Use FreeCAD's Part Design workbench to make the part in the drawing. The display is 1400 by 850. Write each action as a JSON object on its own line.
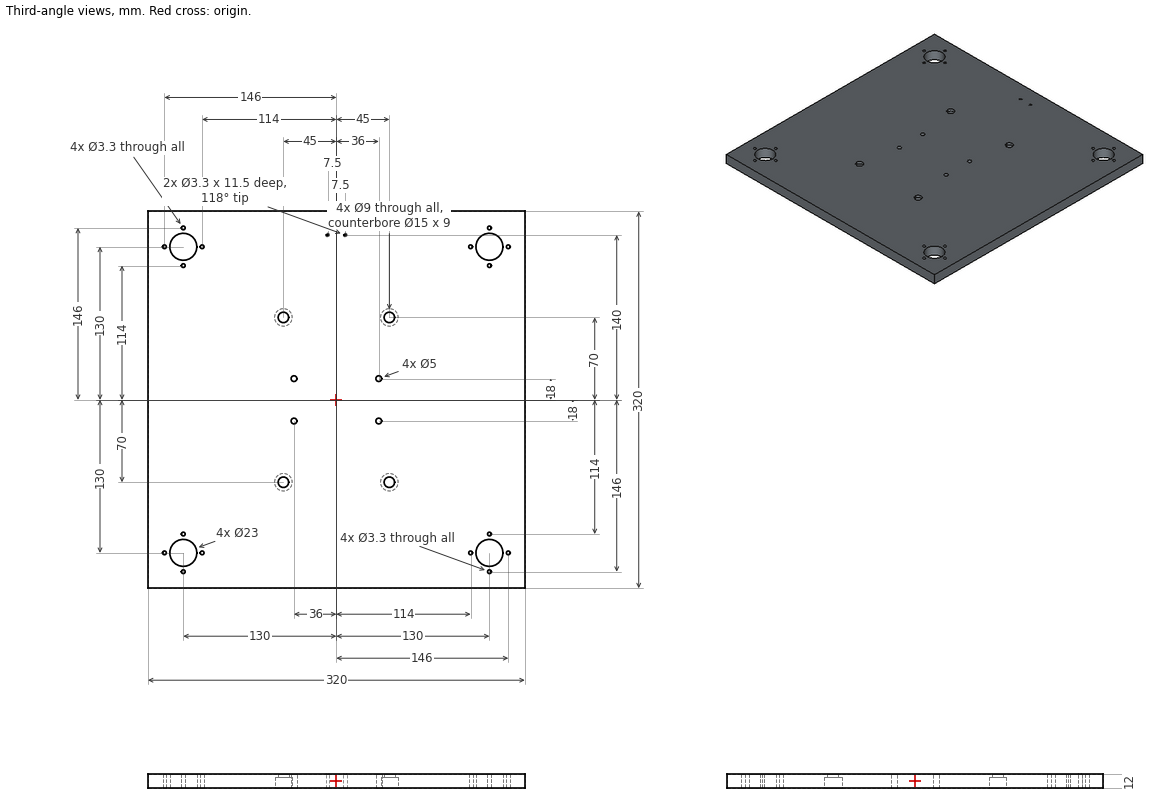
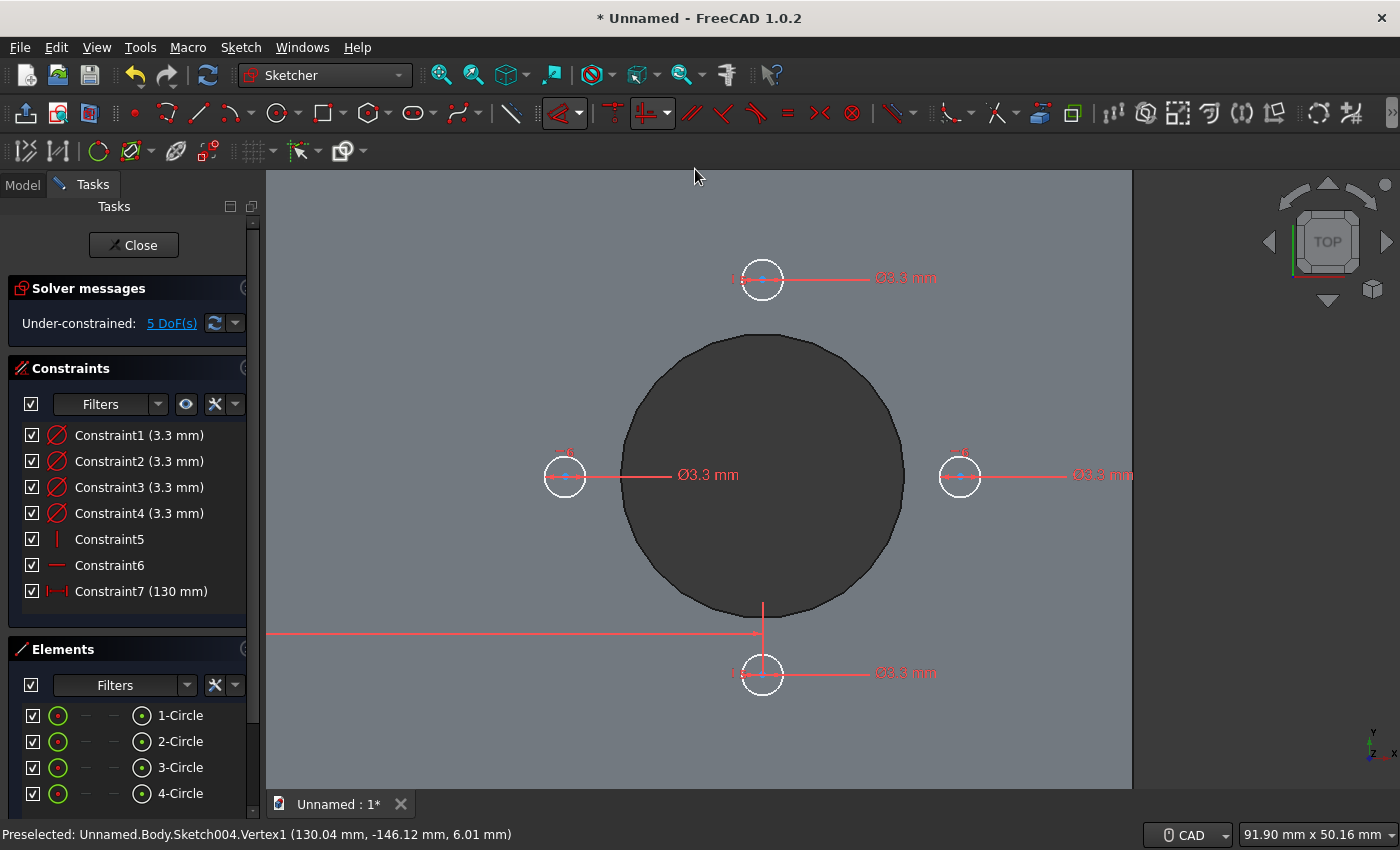
{"action": "left_click", "coordinate": [763, 675]}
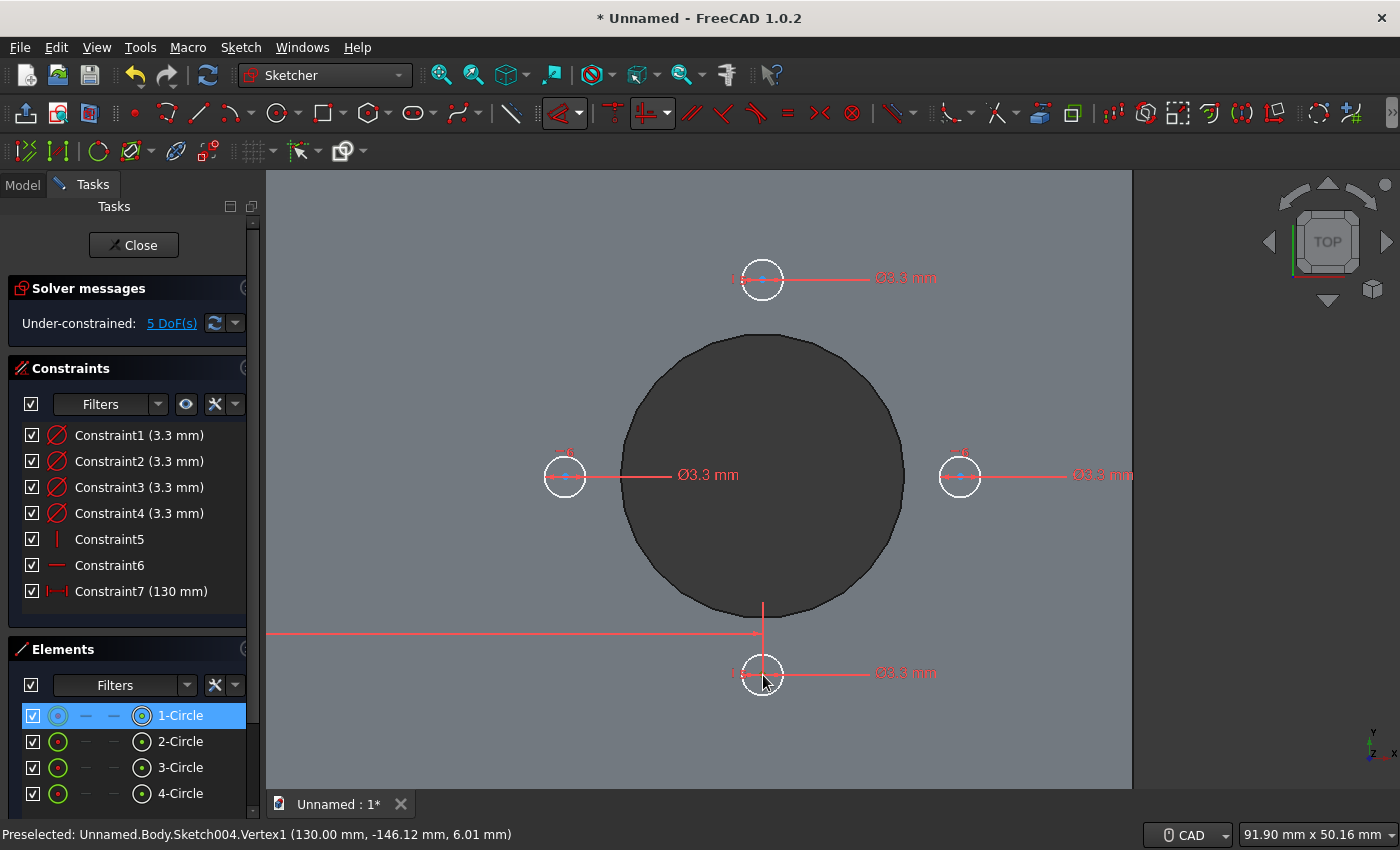
{"action": "left_click", "coordinate": [582, 114]}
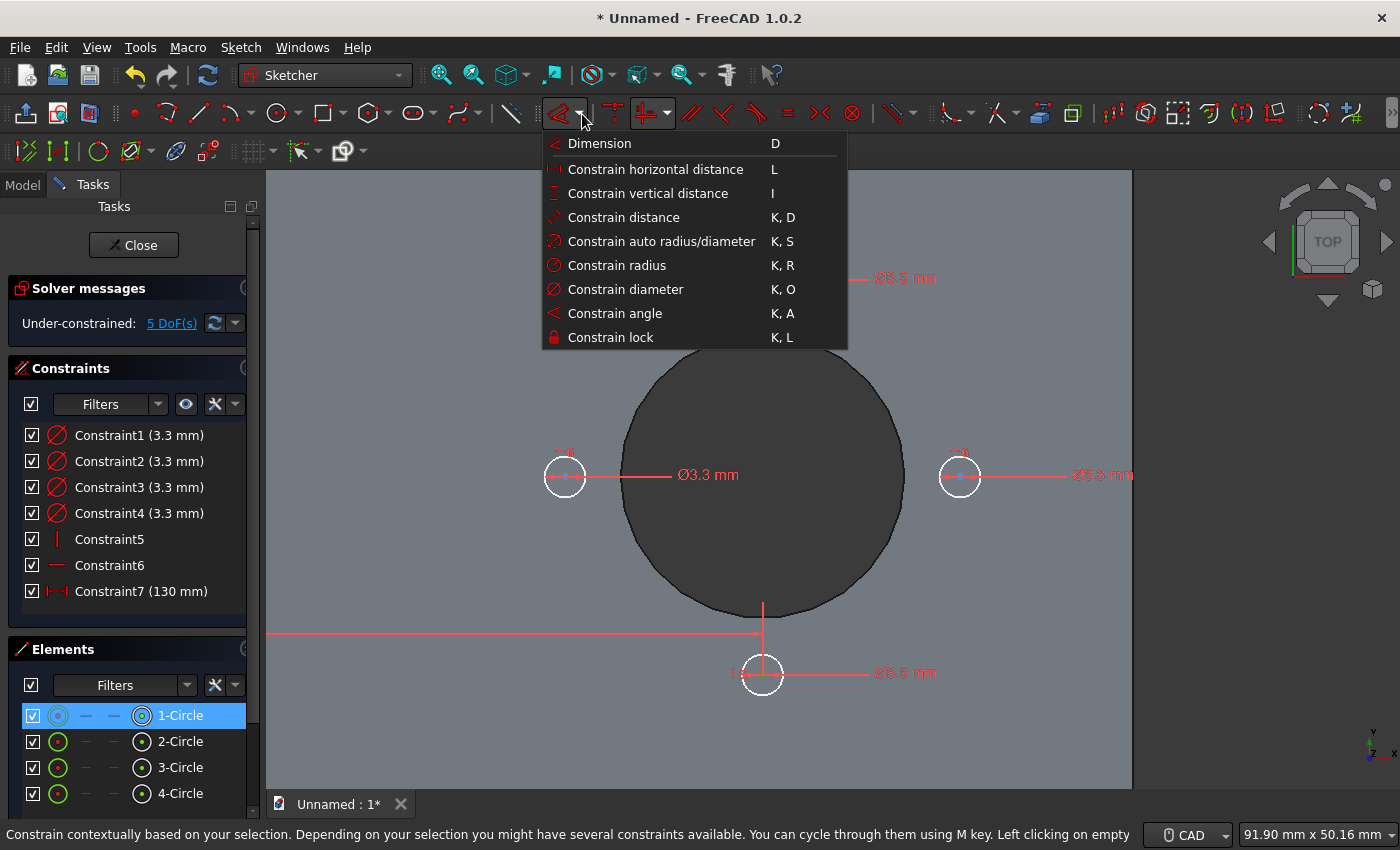
{"action": "left_click", "coordinate": [695, 193]}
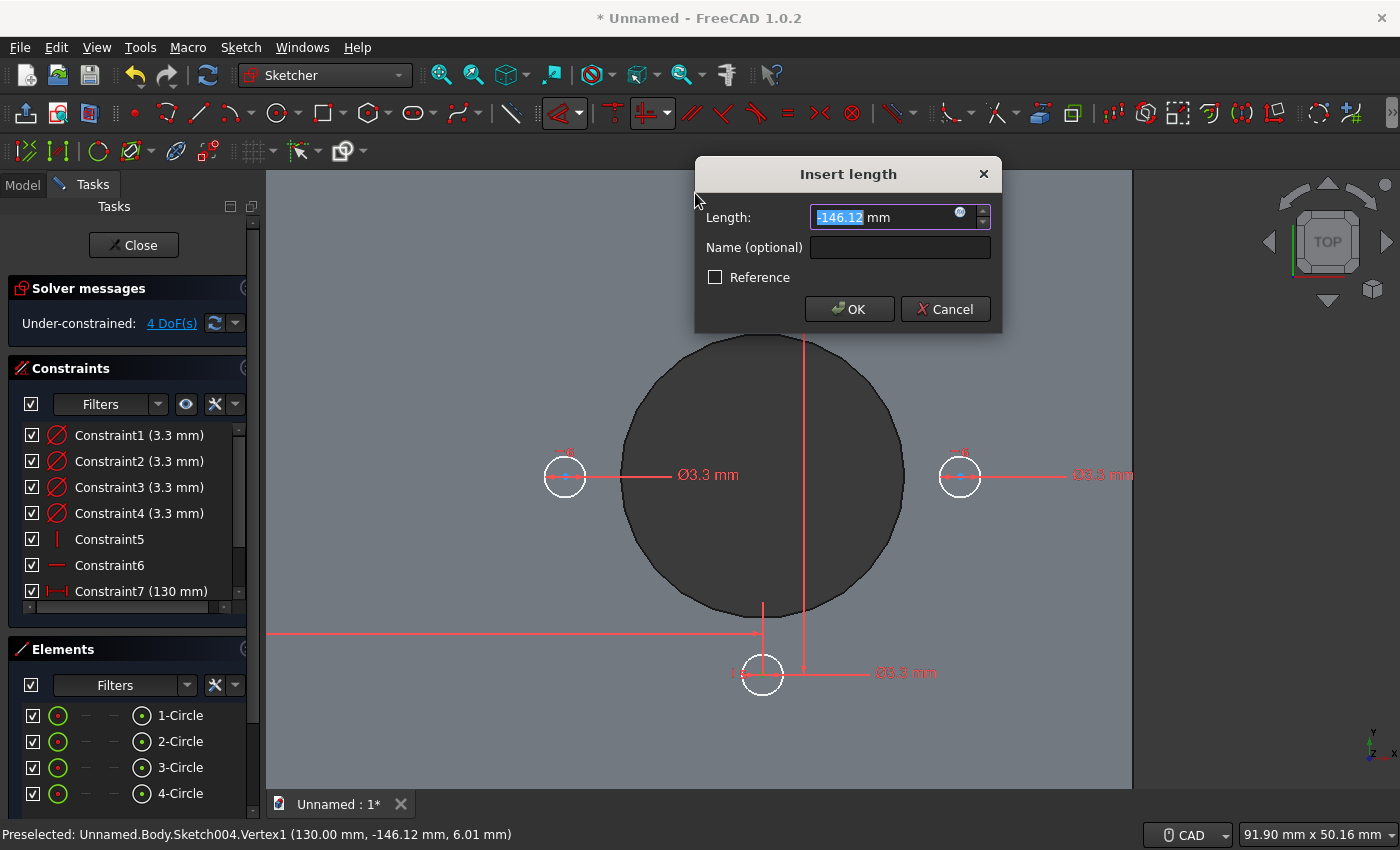
{"action": "type", "text": "-146"}
{"action": "key", "text": "Return"}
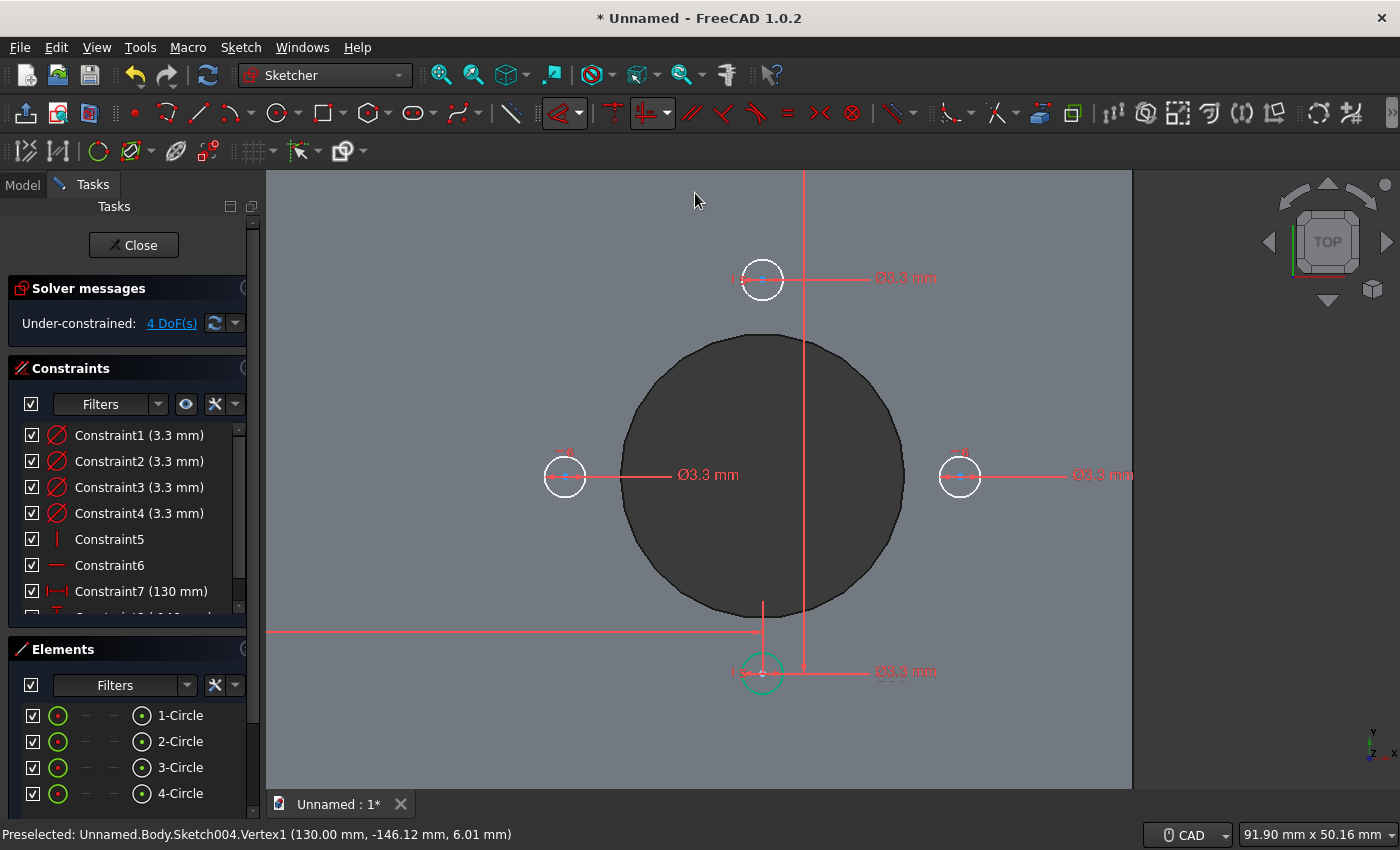
{"action": "left_click", "coordinate": [565, 477]}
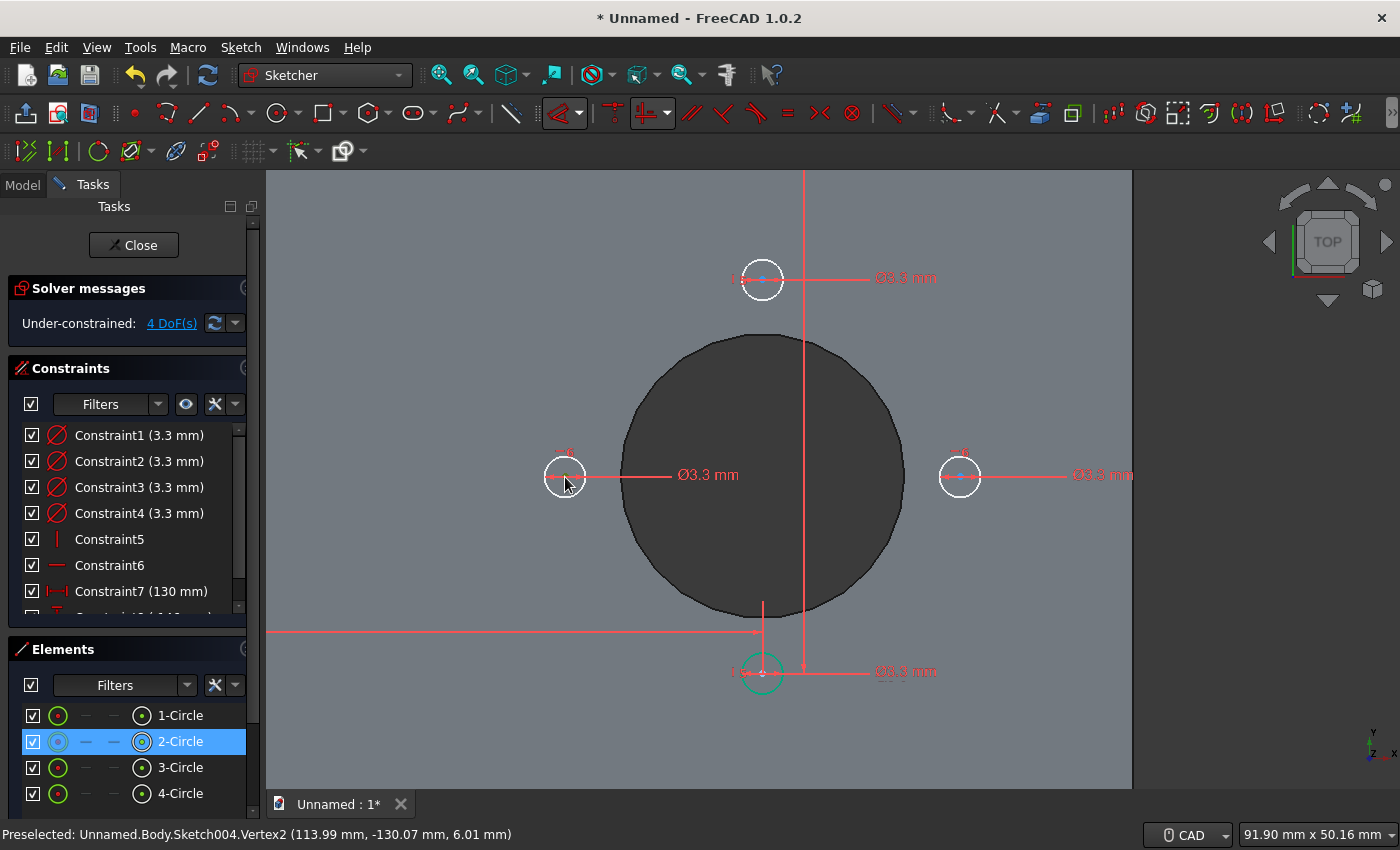
{"action": "left_click", "coordinate": [582, 114]}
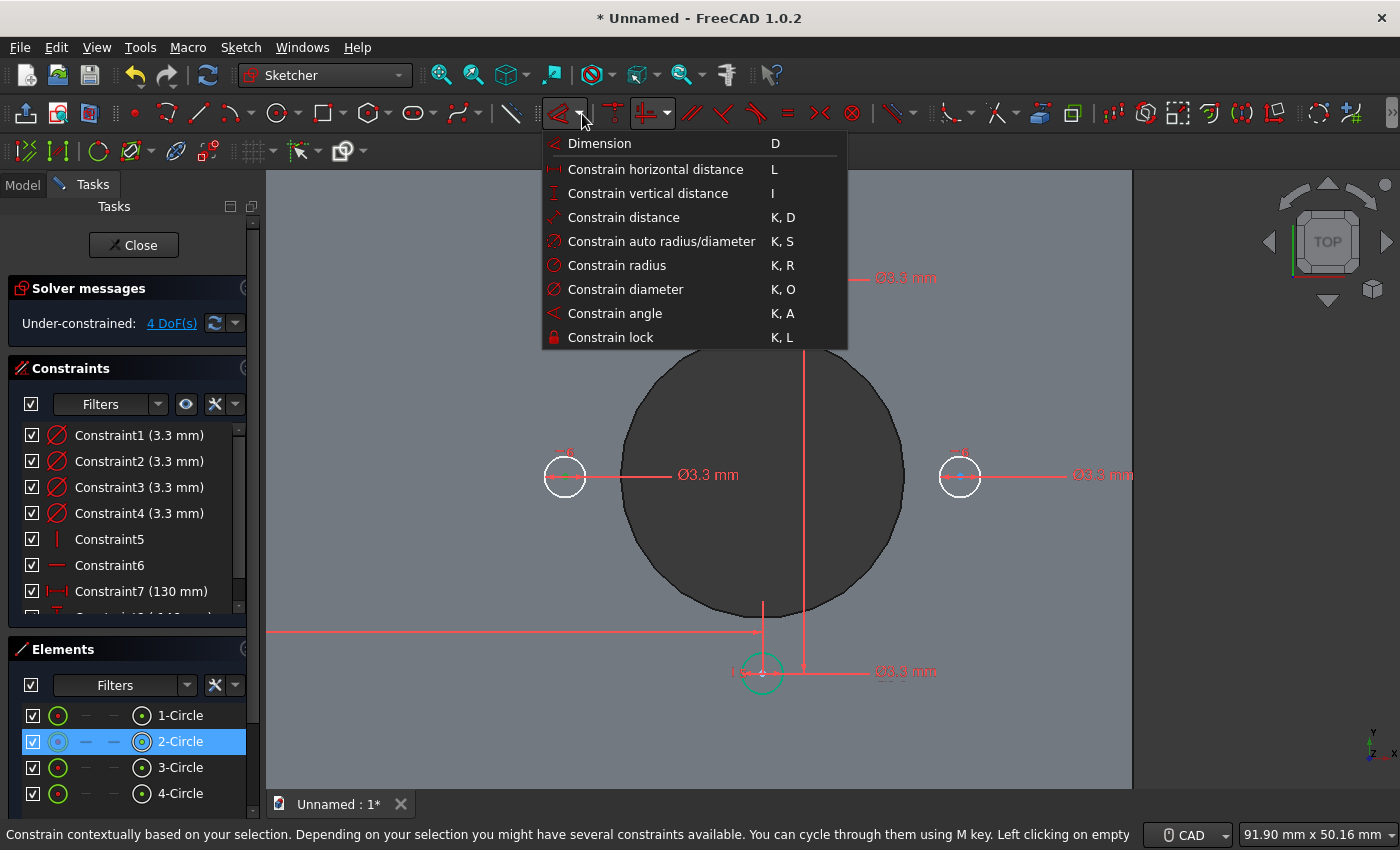
{"action": "left_click", "coordinate": [695, 169]}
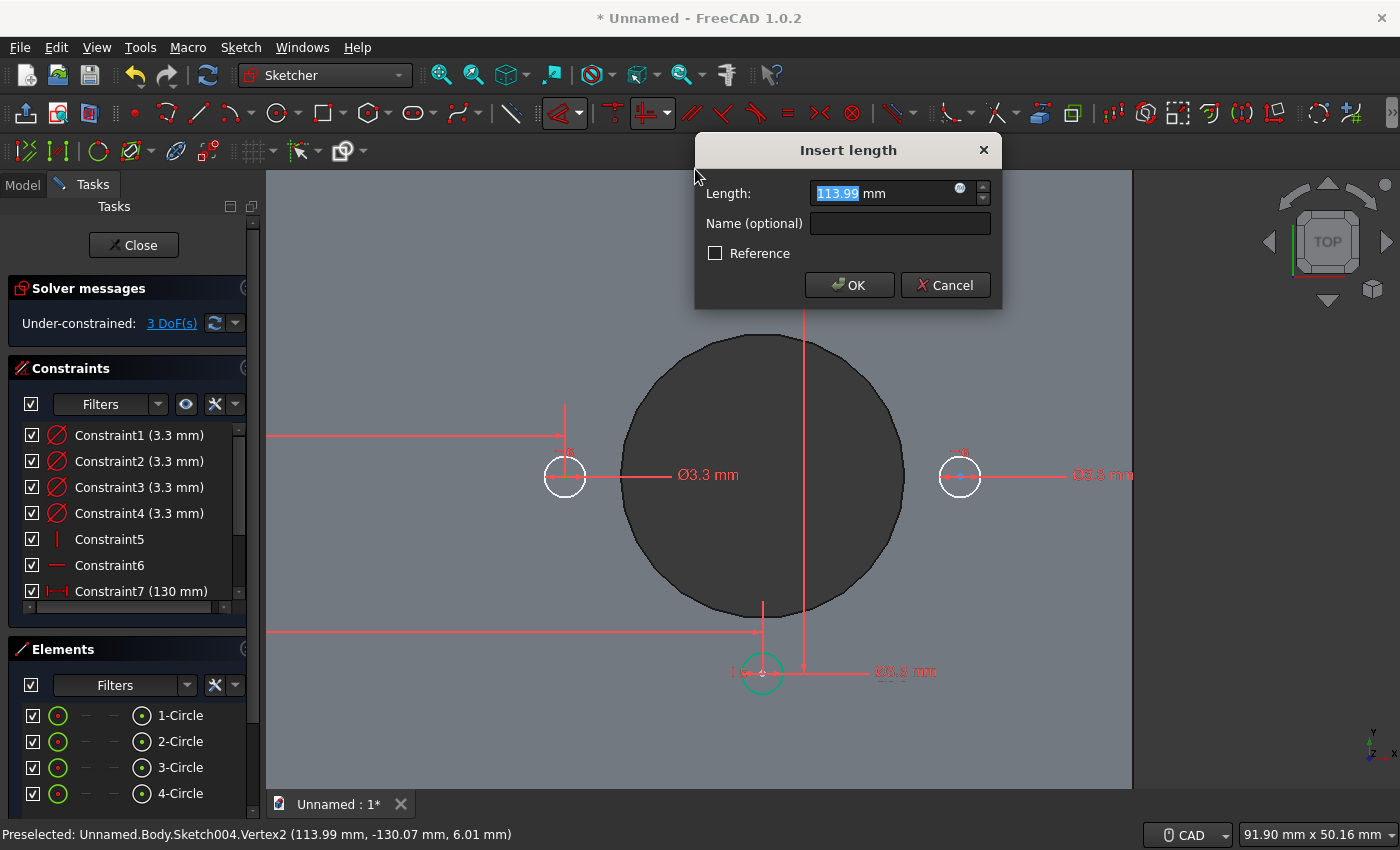
{"action": "type", "text": "114"}
{"action": "key", "text": "Return"}